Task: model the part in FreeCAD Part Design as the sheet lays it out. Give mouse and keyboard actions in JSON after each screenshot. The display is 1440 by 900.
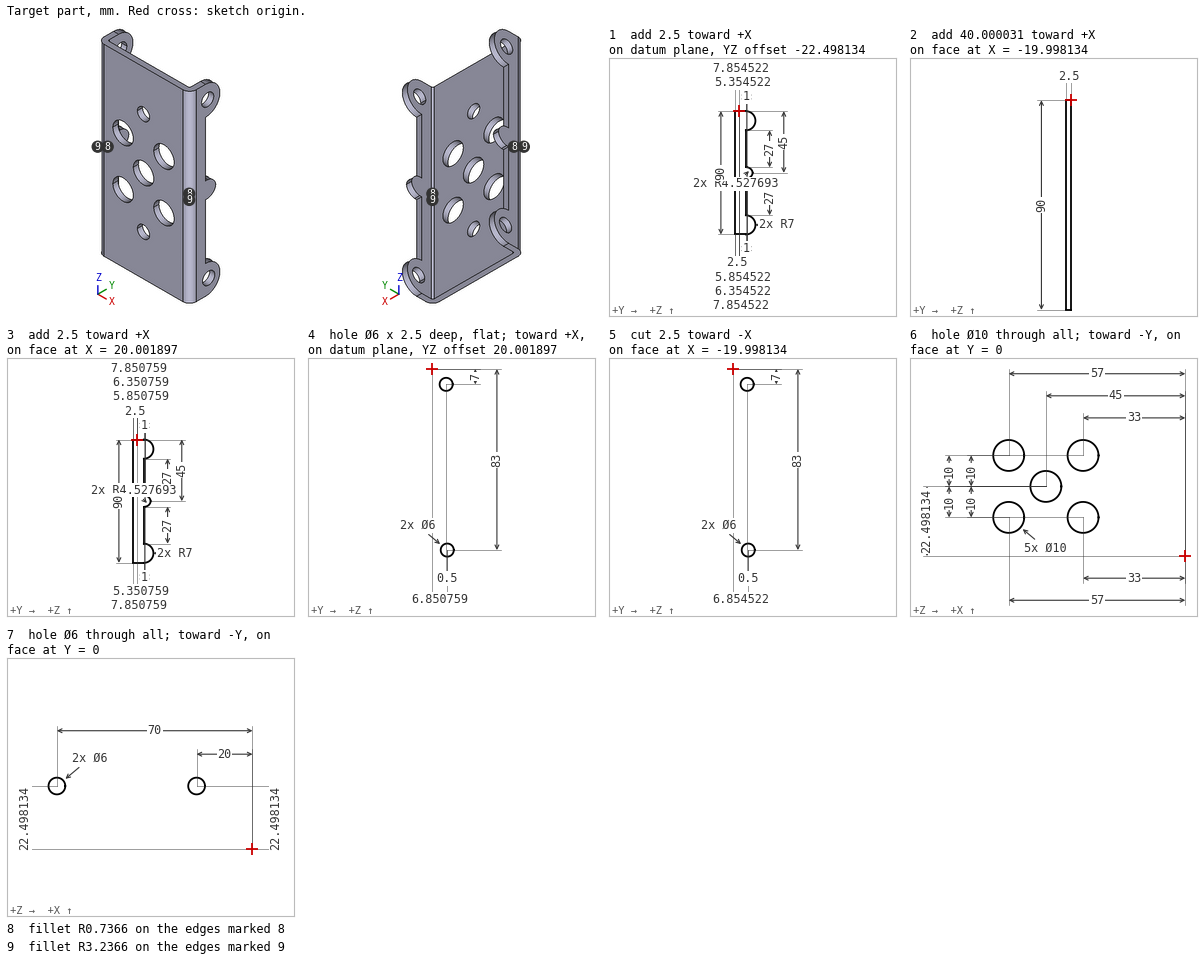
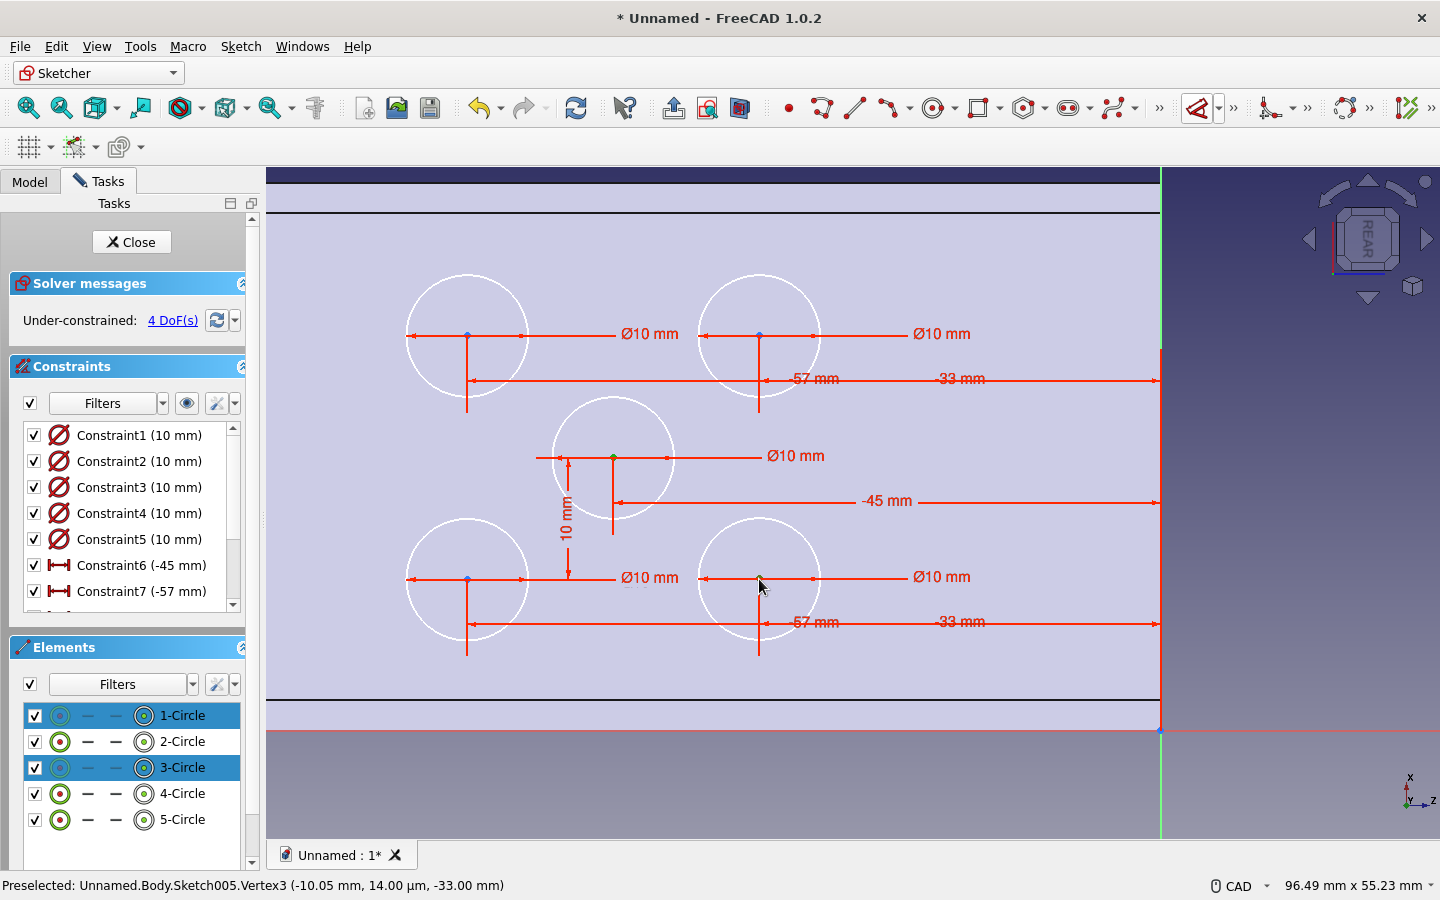
{"action": "key", "text": "i"}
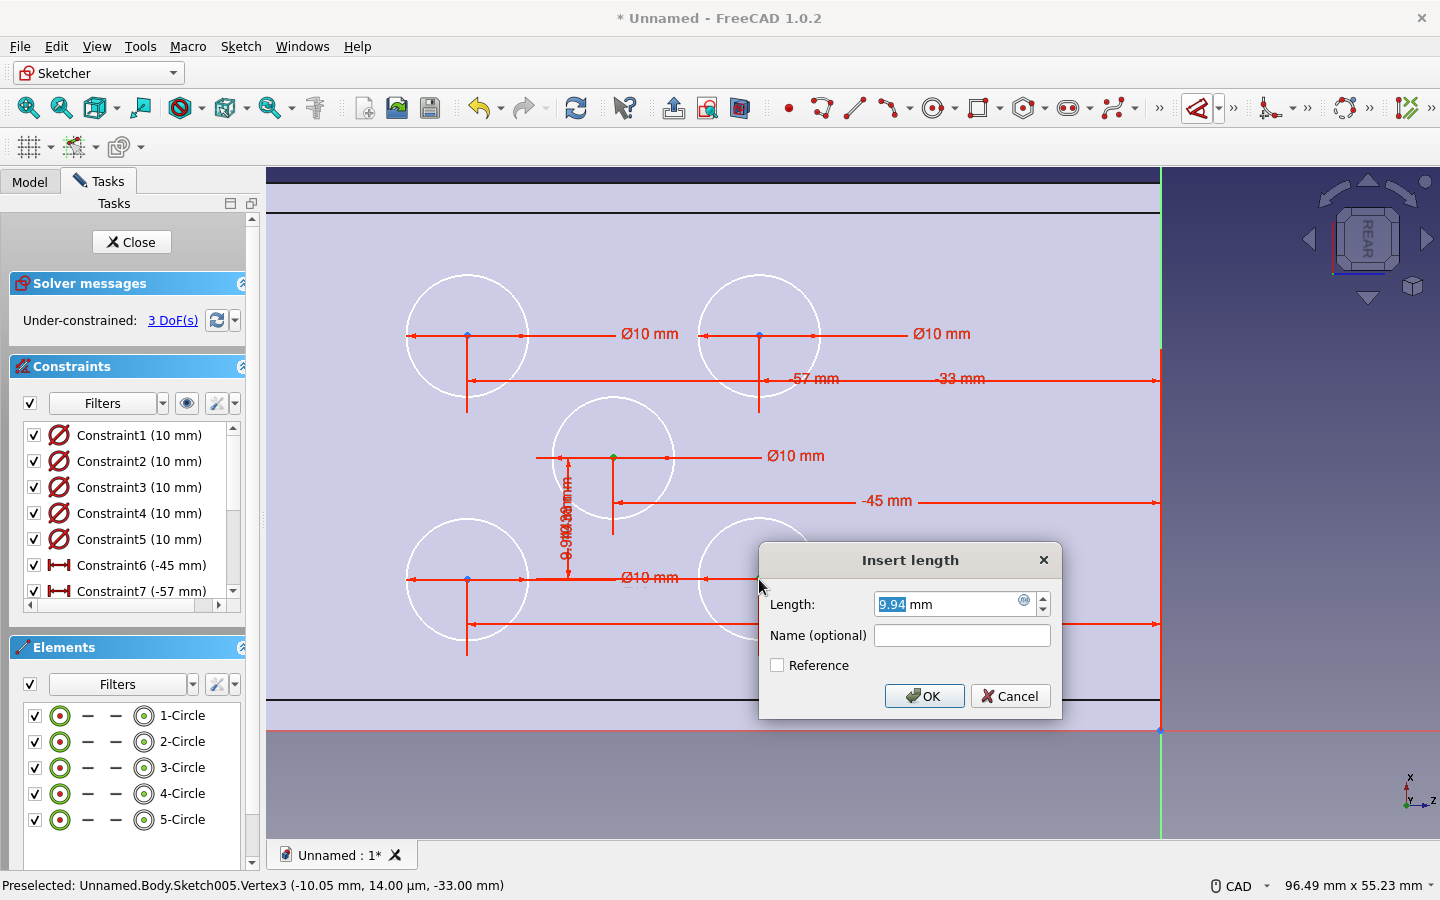
{"action": "type", "text": "10"}
{"action": "key", "text": "Return"}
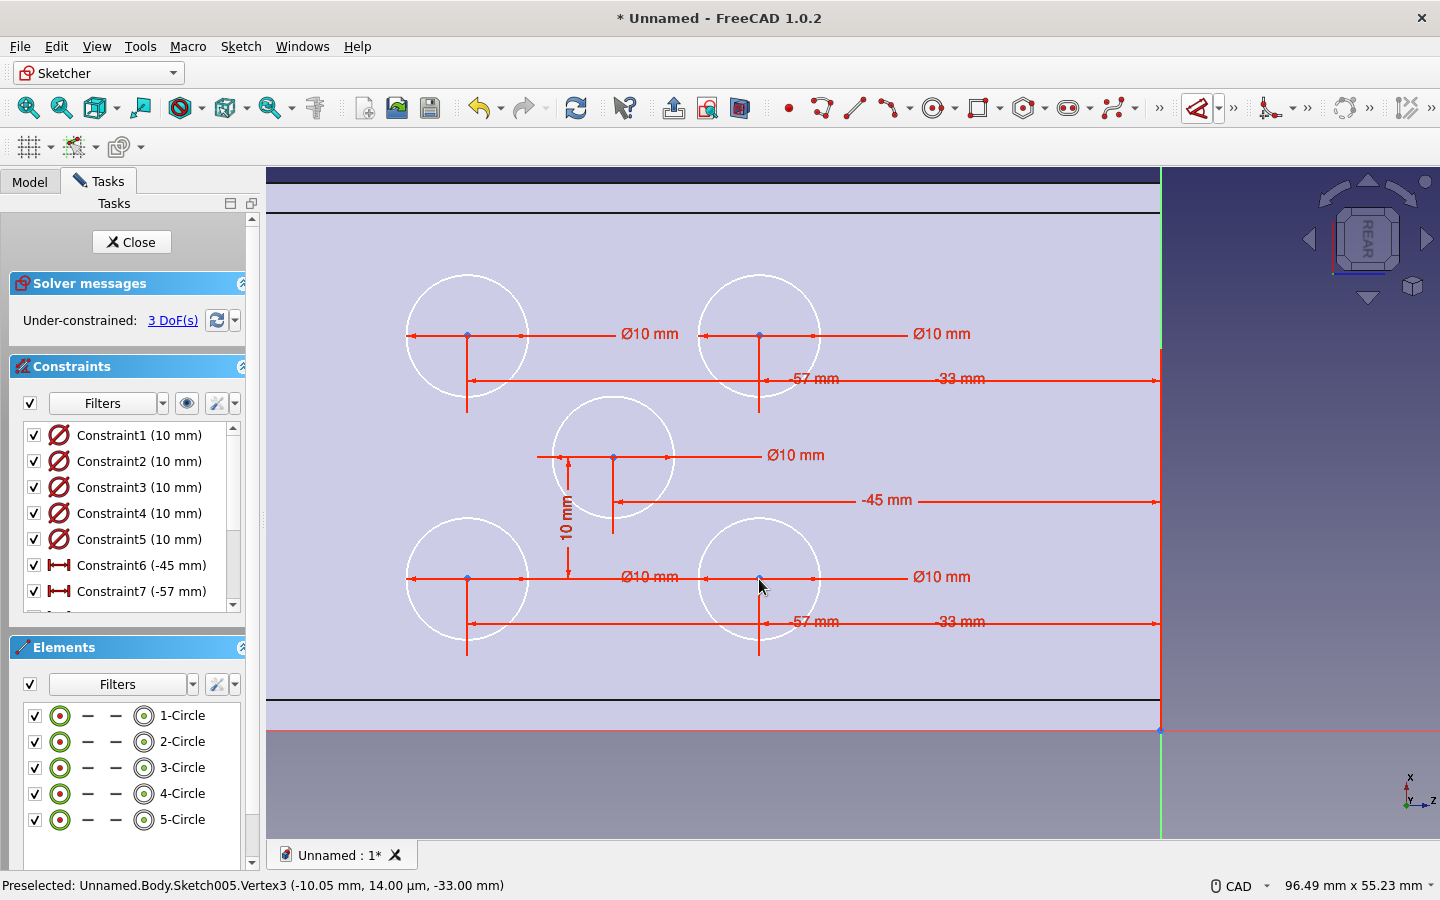
{"action": "left_click", "coordinate": [613, 457]}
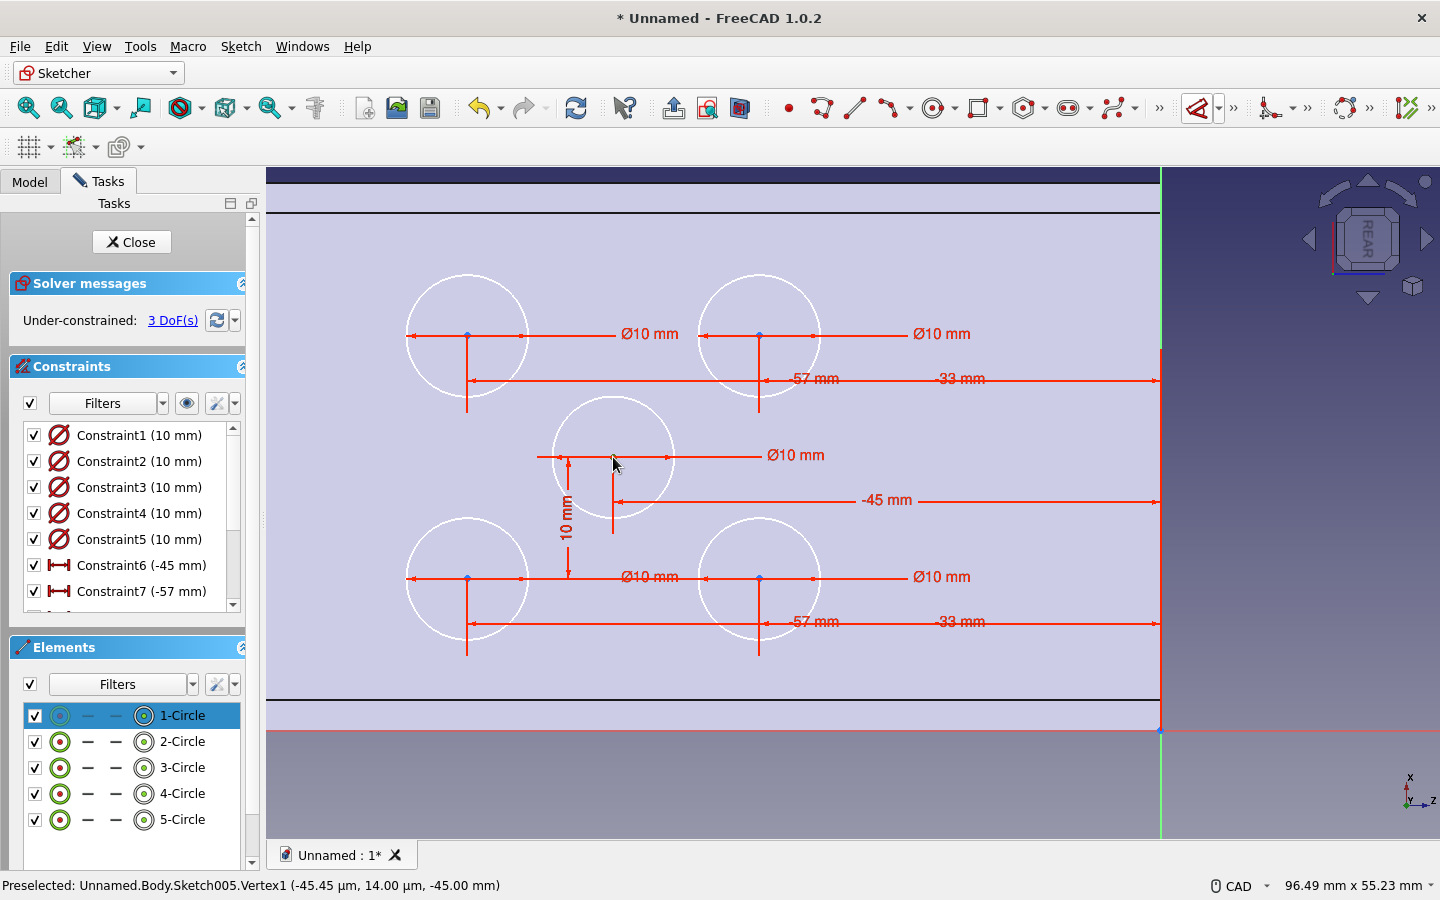
{"action": "left_click", "coordinate": [759, 336]}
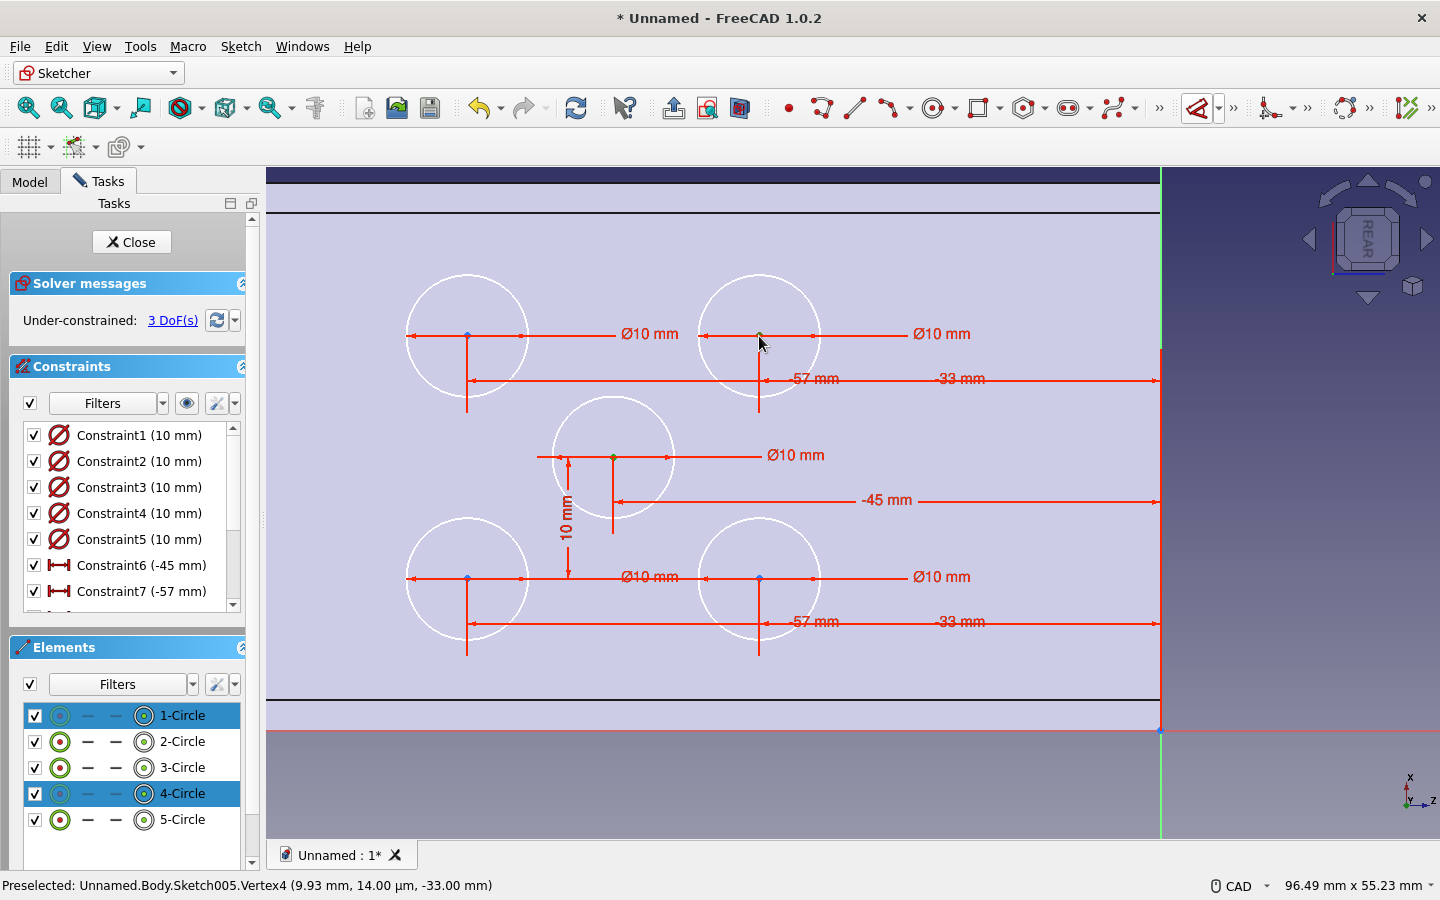
{"action": "key", "text": "i"}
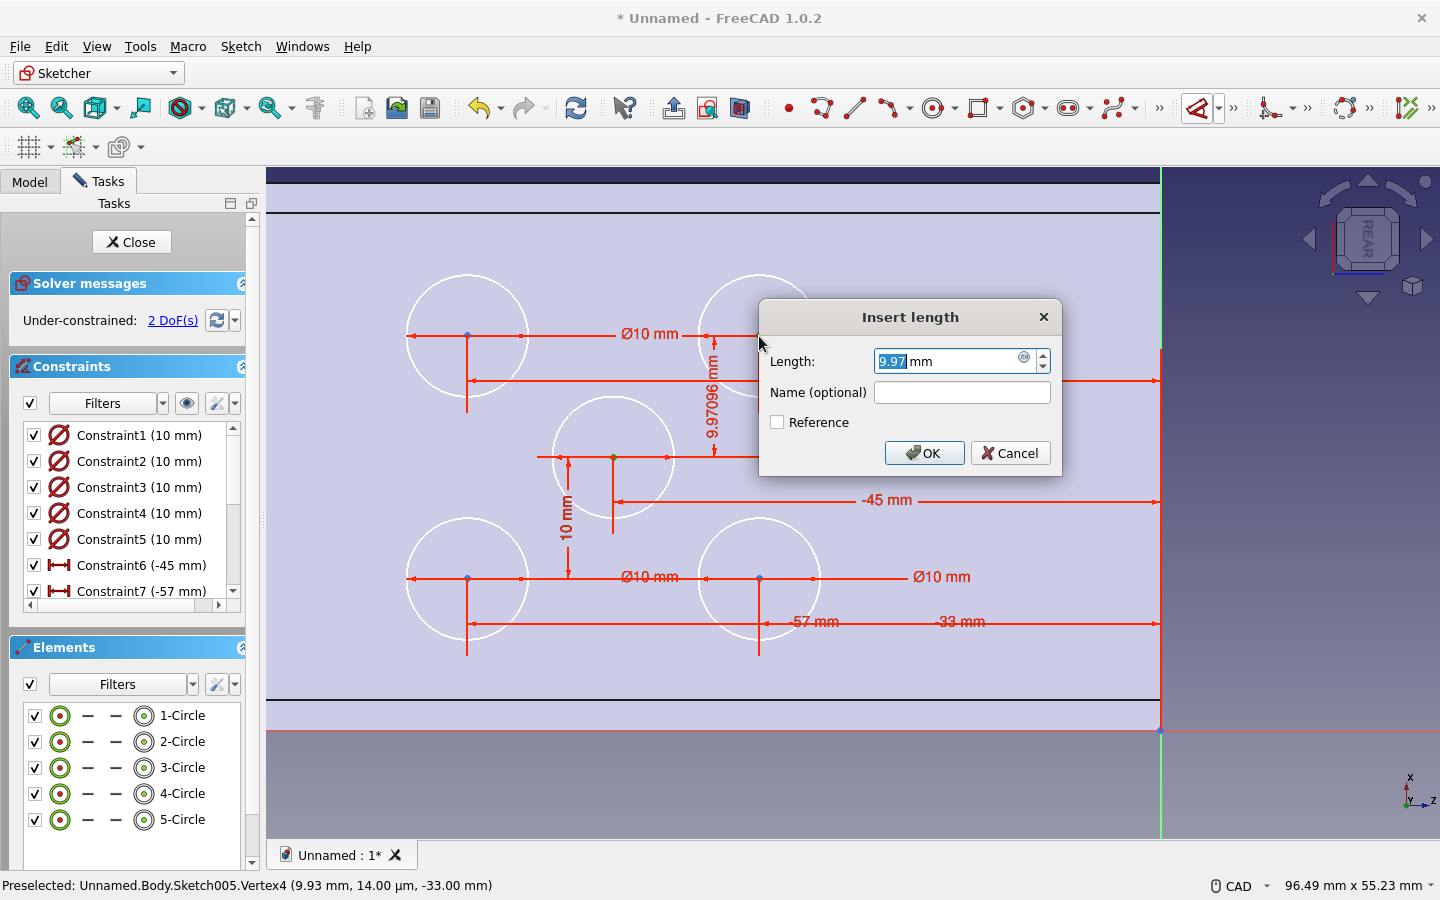
{"action": "type", "text": "10"}
{"action": "key", "text": "Return"}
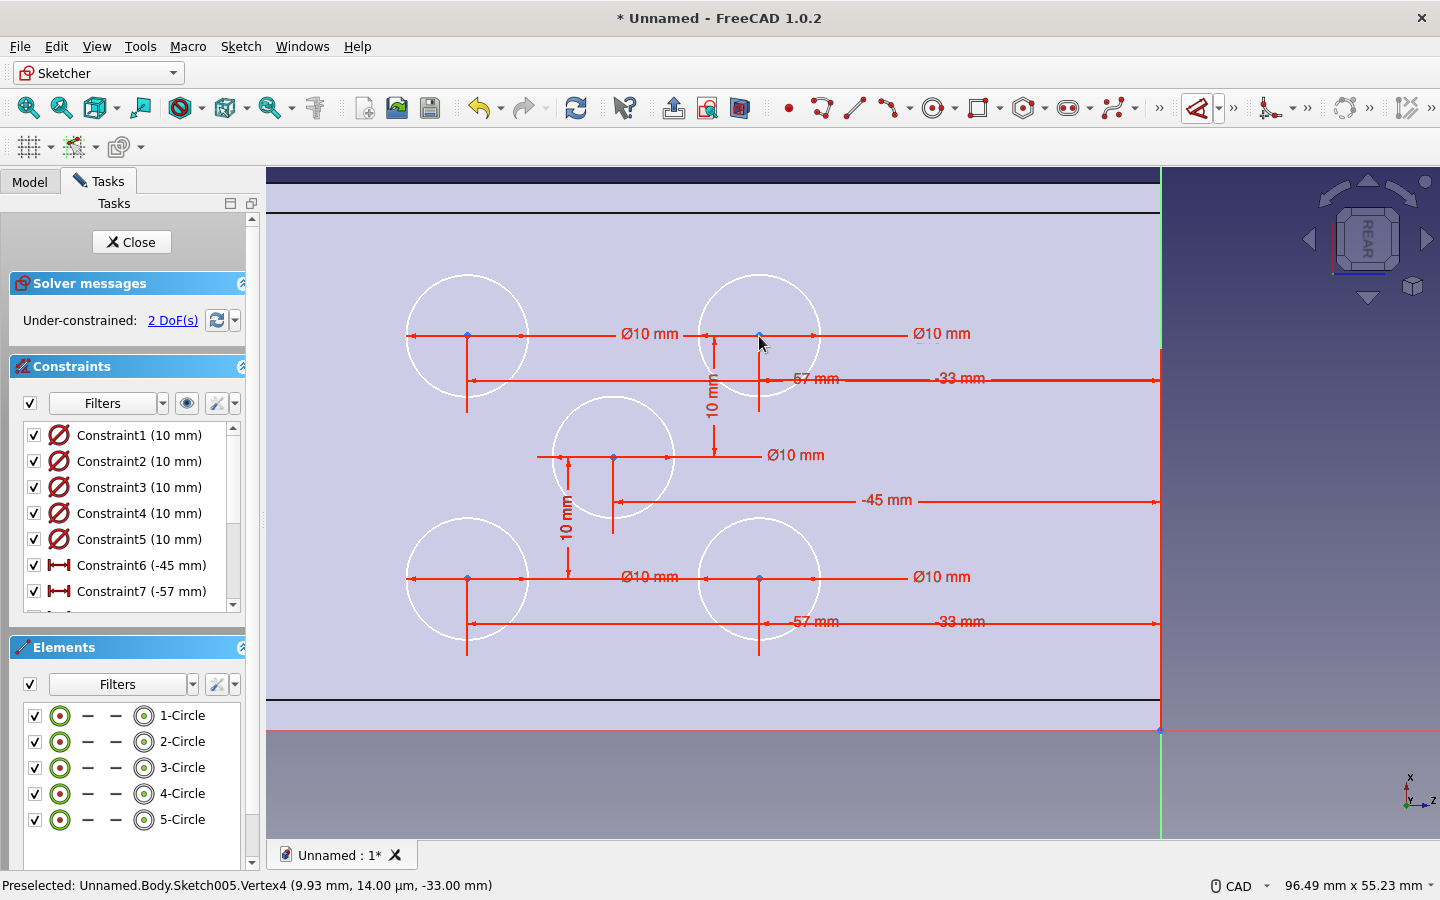
{"action": "left_click", "coordinate": [613, 457]}